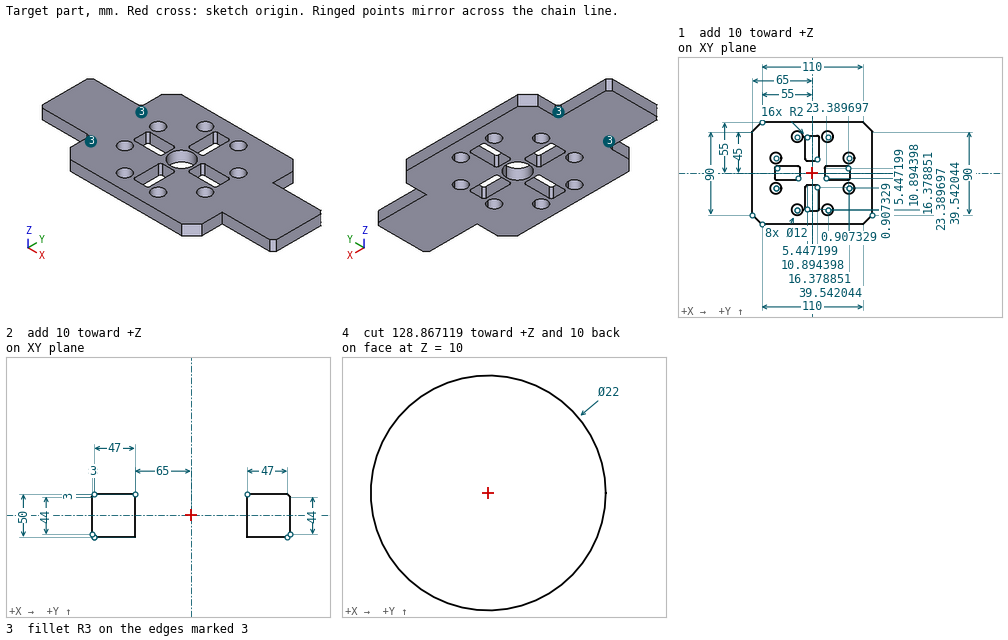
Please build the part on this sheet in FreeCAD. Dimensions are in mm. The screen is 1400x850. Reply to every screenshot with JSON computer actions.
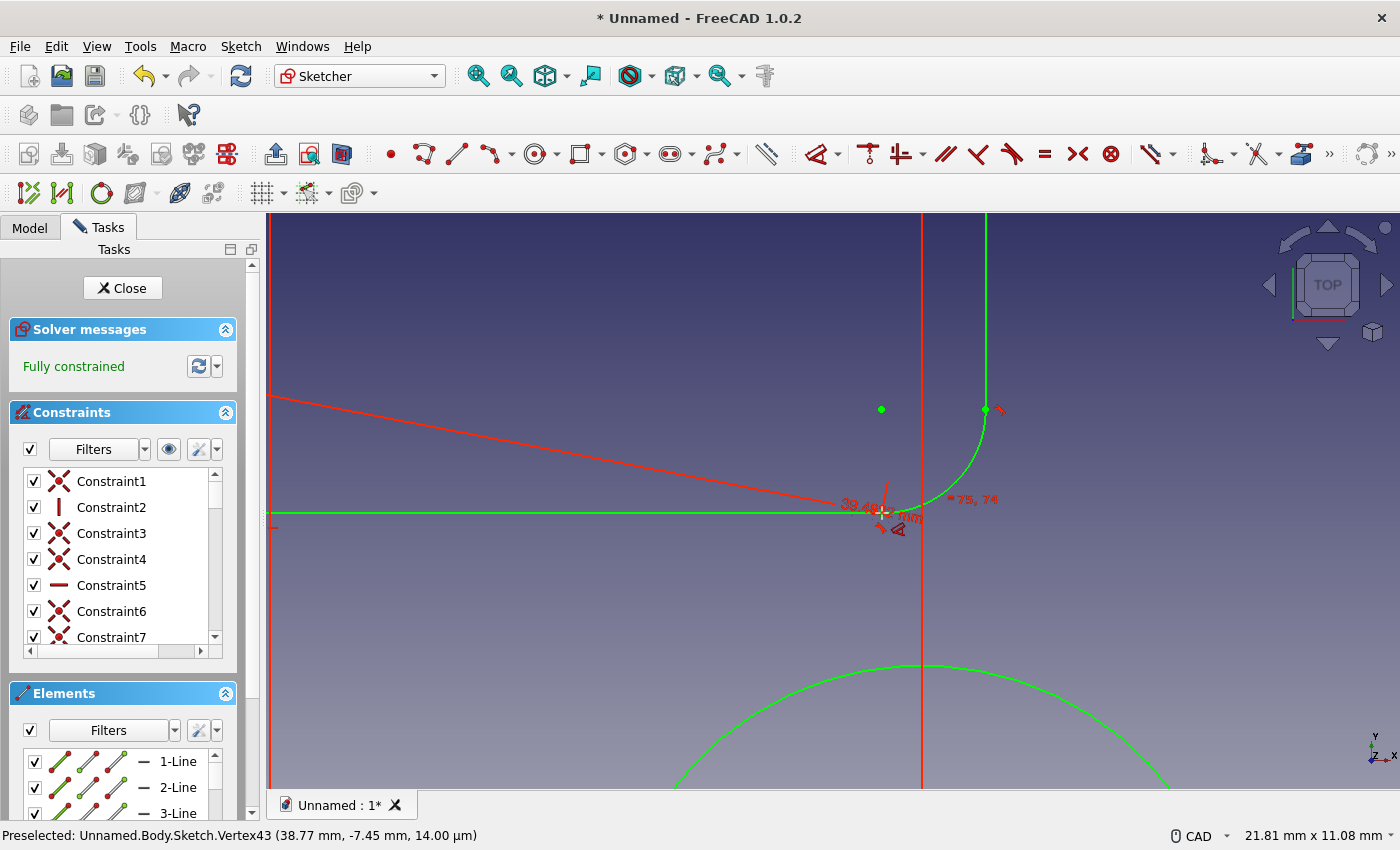
{"action": "scroll", "coordinate": [887, 525], "scroll_direction": "down", "scroll_amount": 14}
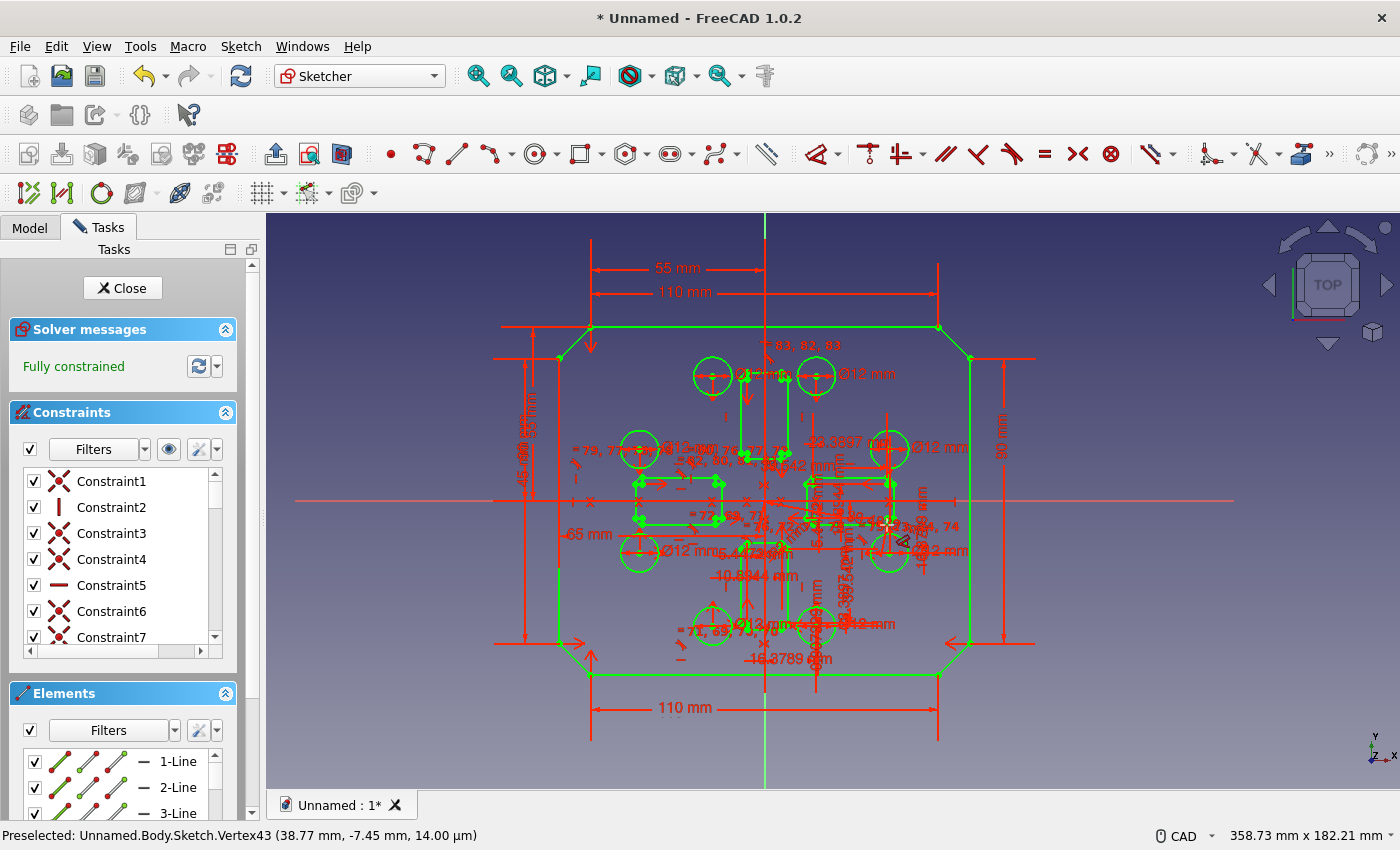
{"action": "scroll", "coordinate": [890, 553], "scroll_direction": "up", "scroll_amount": 14}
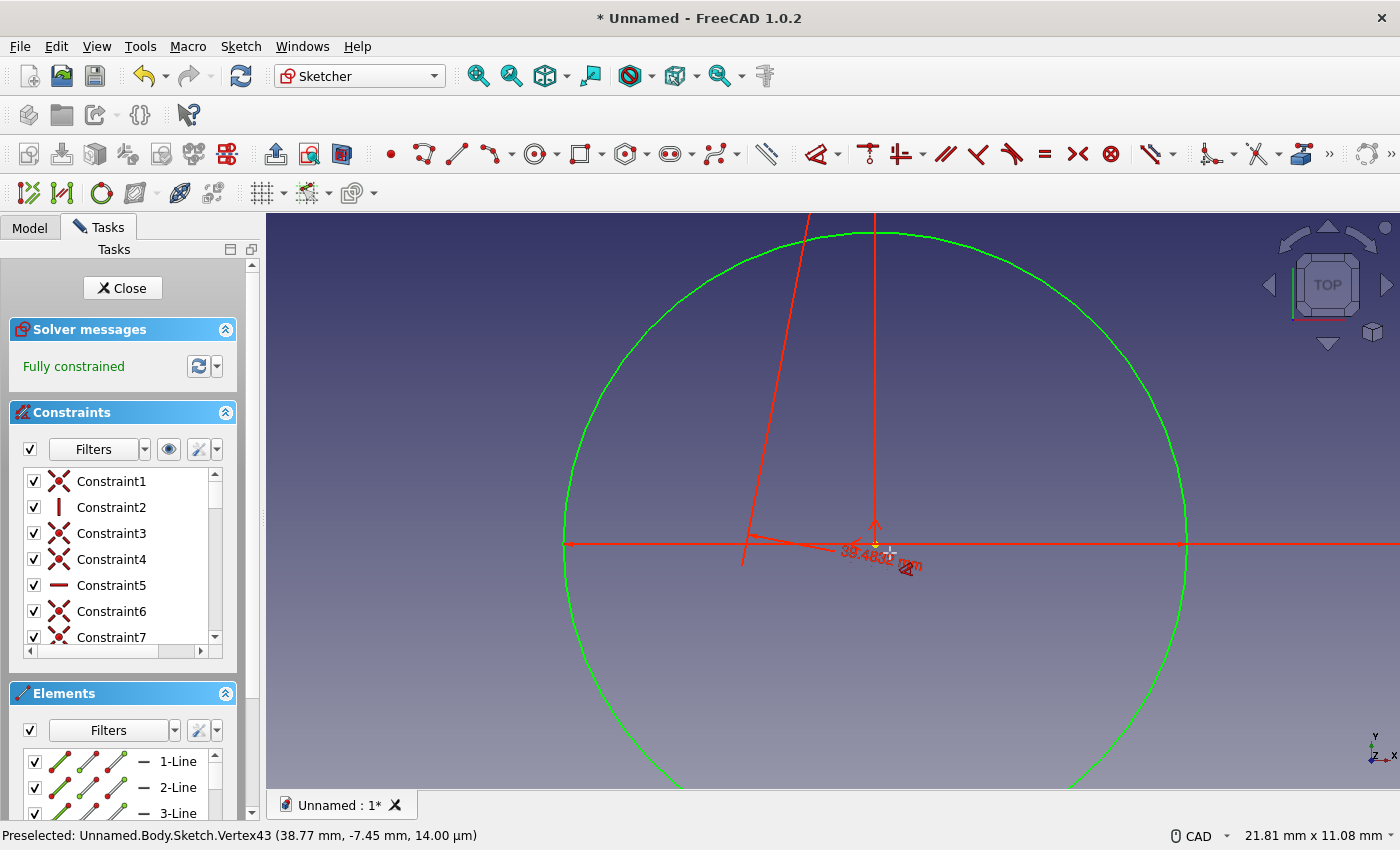
{"action": "left_click", "coordinate": [875, 544]}
{"action": "left_click", "coordinate": [855, 578]}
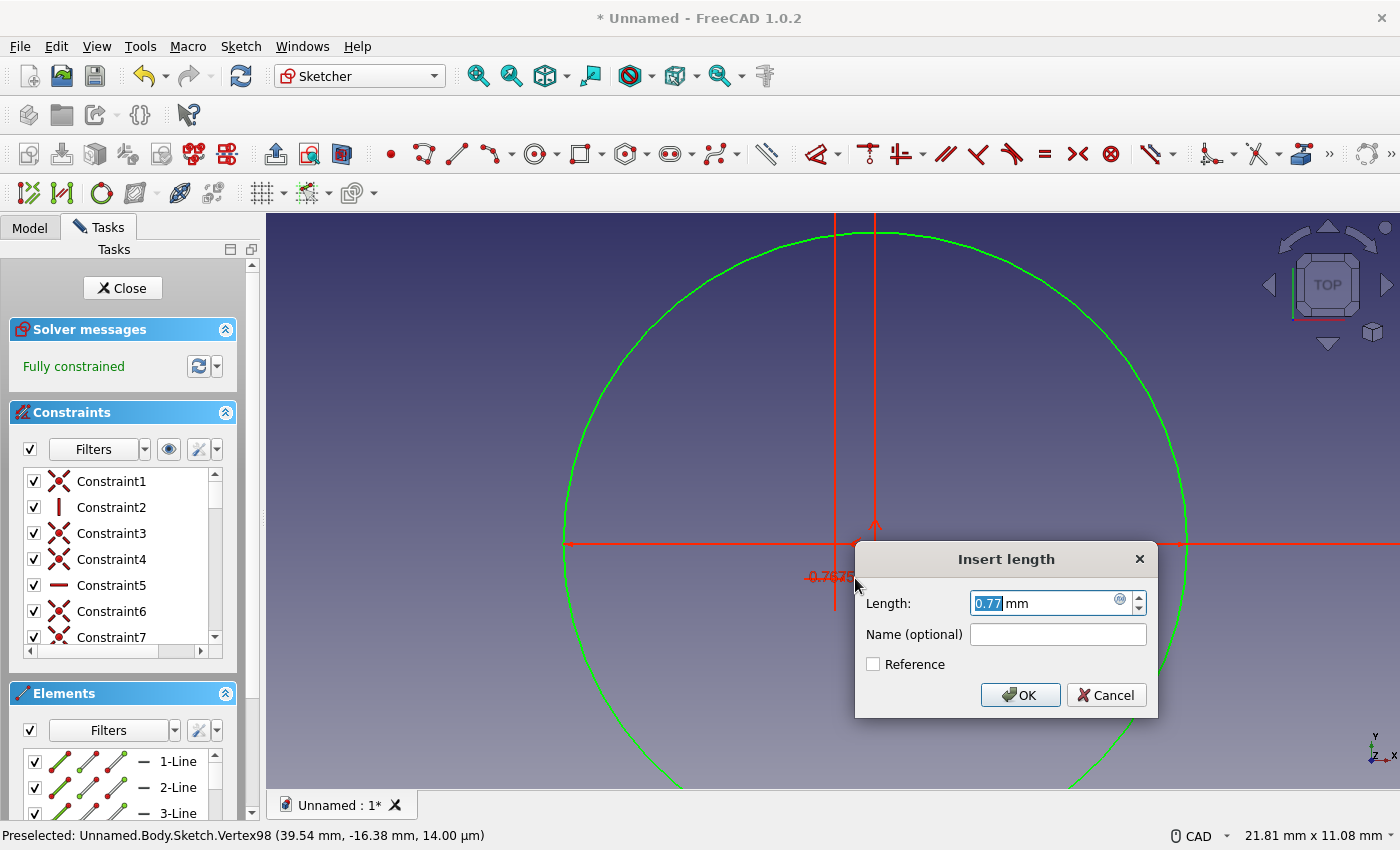
{"action": "type", "text": "0.907329"}
{"action": "key", "text": "Return"}
{"action": "key", "text": "Escape"}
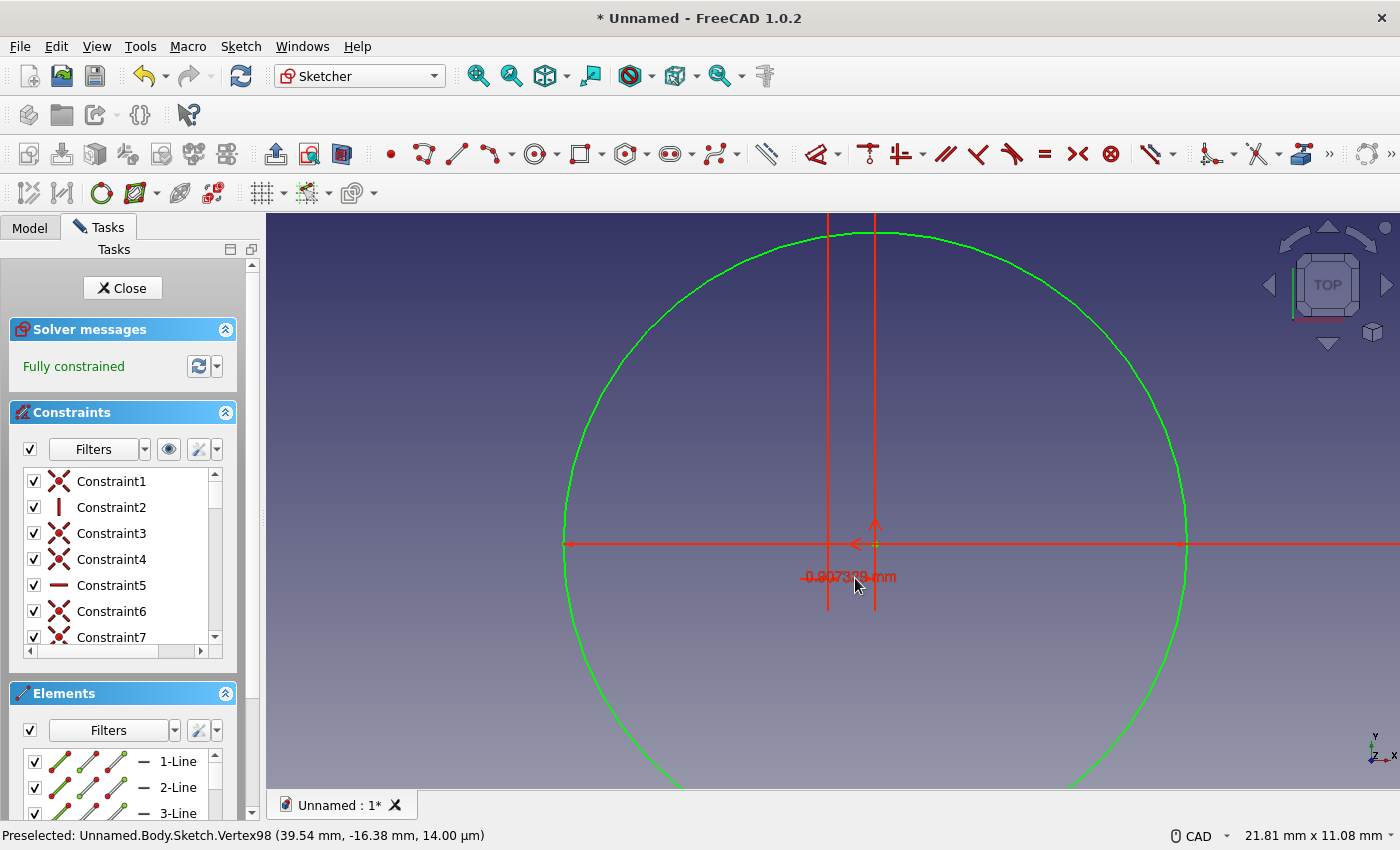
{"action": "left_click", "coordinate": [123, 288]}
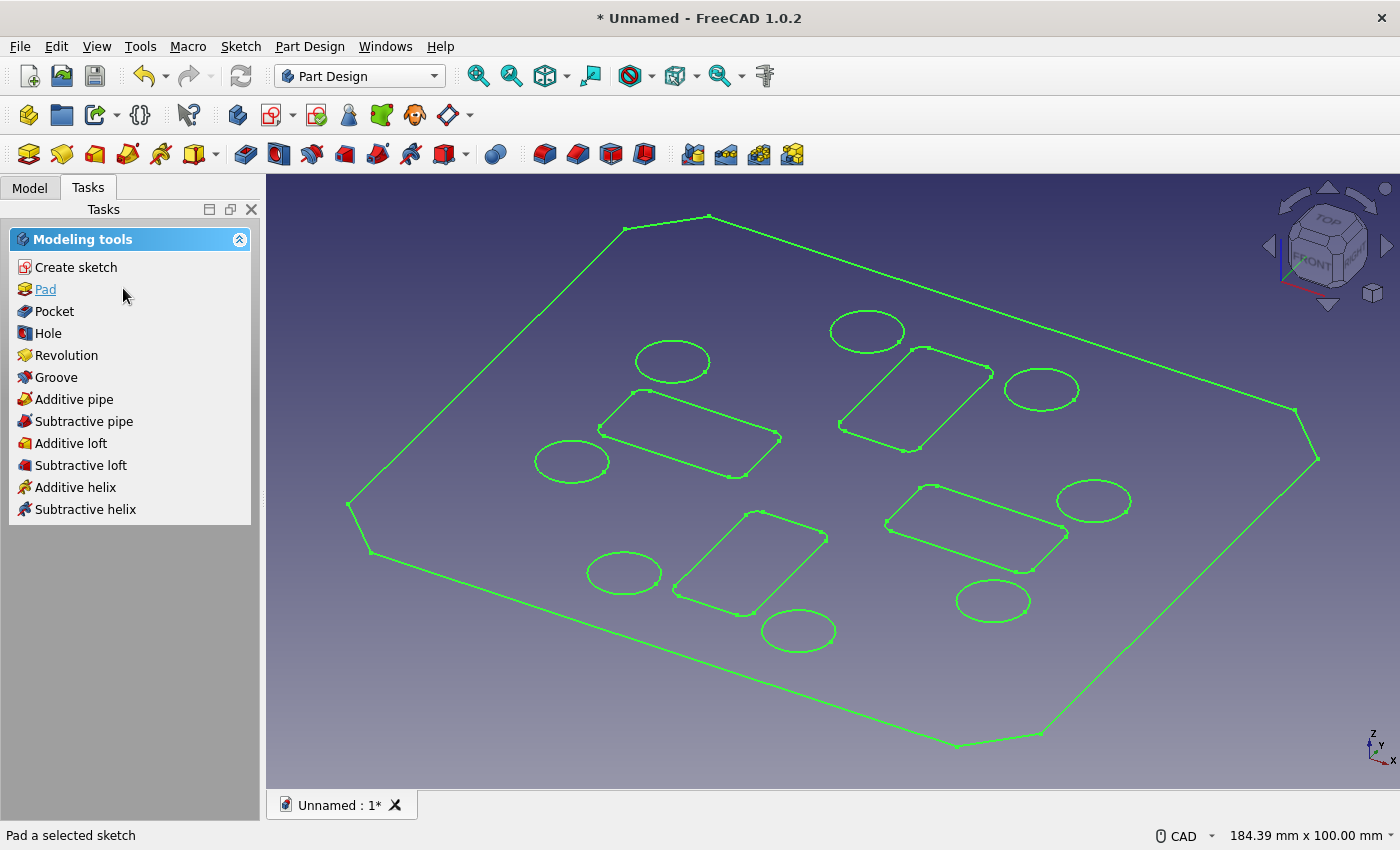
{"action": "left_click", "coordinate": [29, 154]}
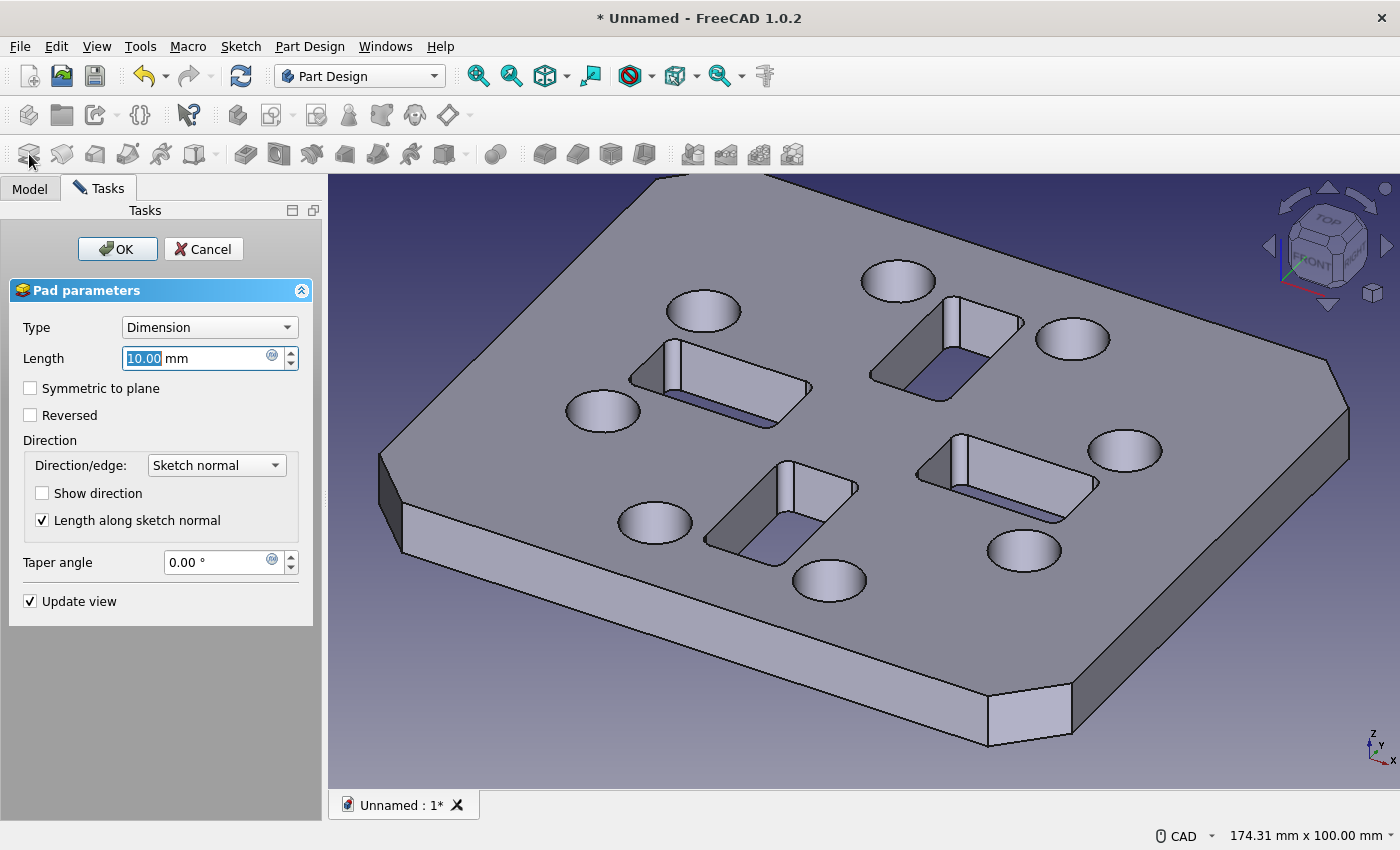
{"action": "type", "text": "10"}
{"action": "key", "text": "Tab"}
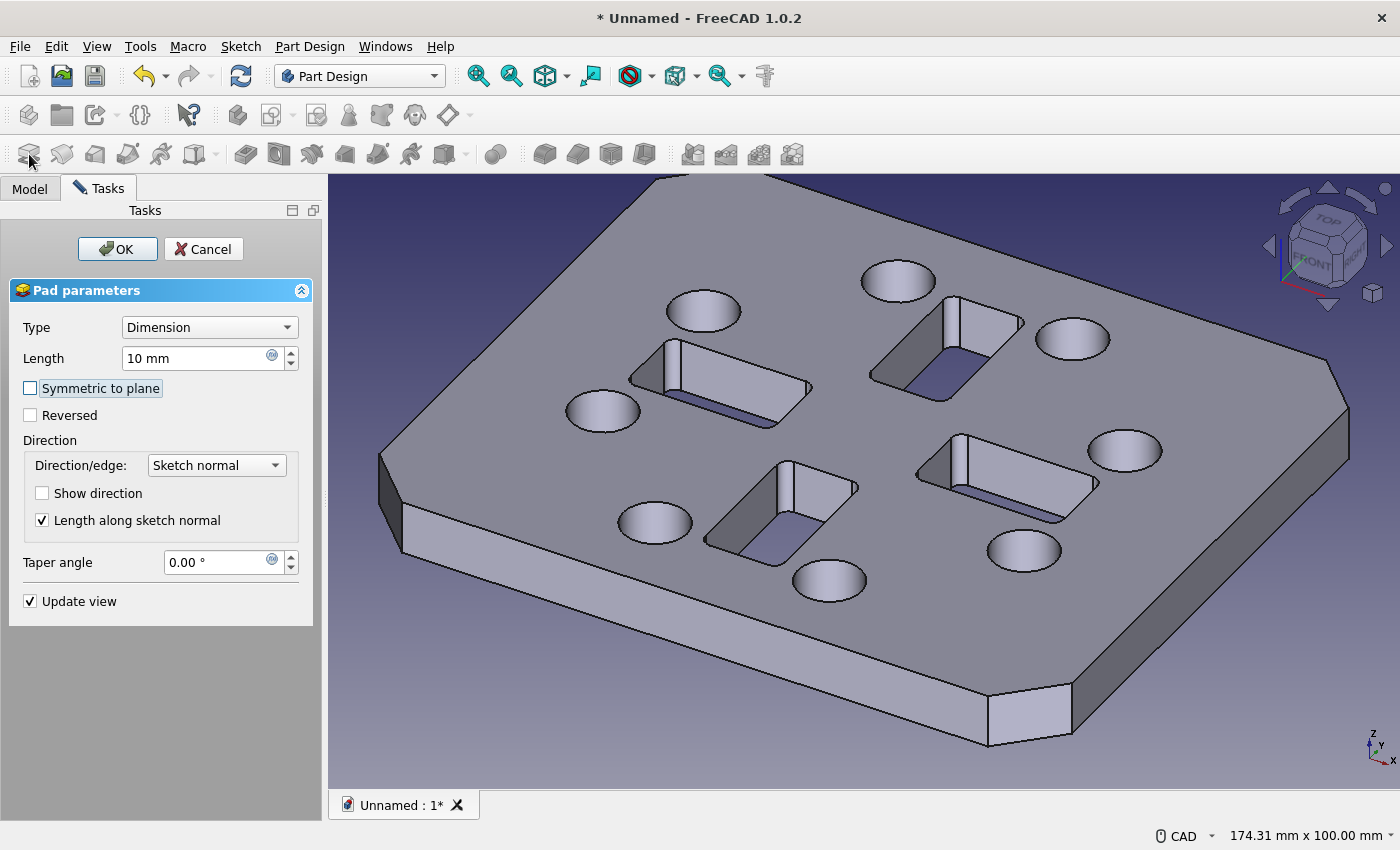
{"action": "left_click", "coordinate": [118, 249]}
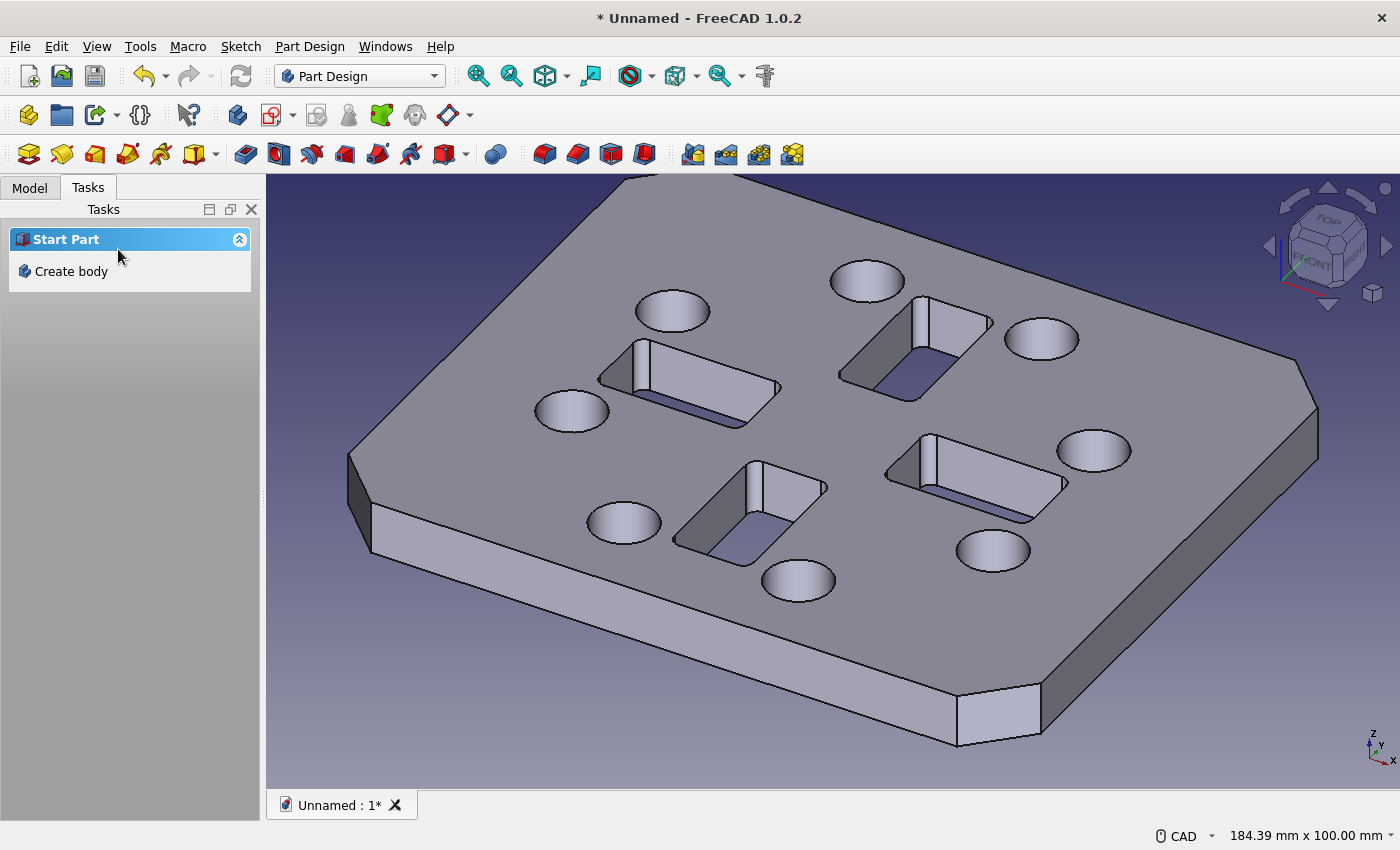
{"action": "left_click", "coordinate": [479, 76]}